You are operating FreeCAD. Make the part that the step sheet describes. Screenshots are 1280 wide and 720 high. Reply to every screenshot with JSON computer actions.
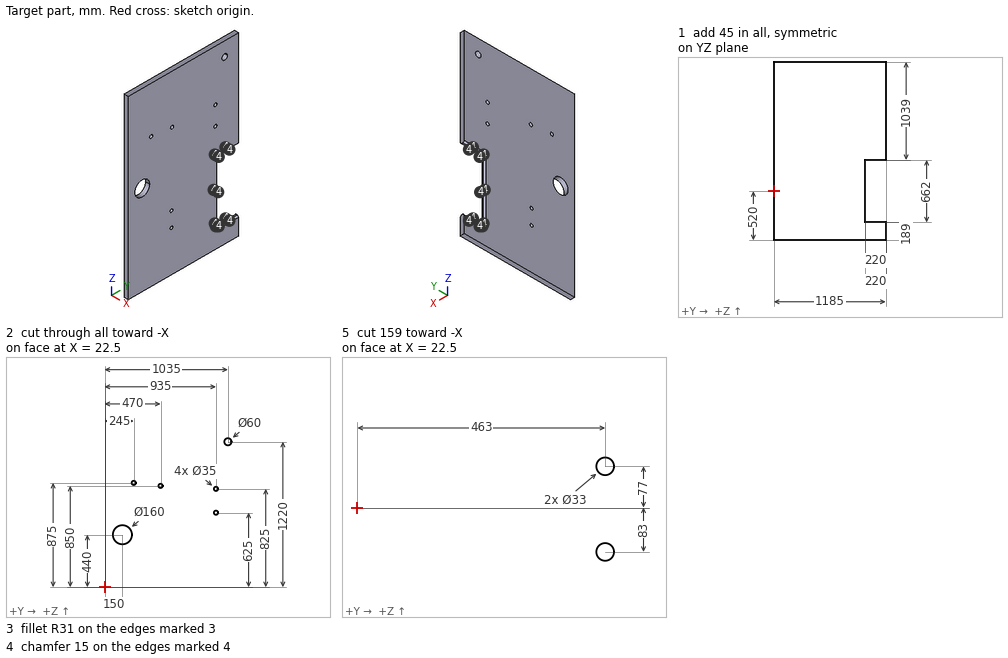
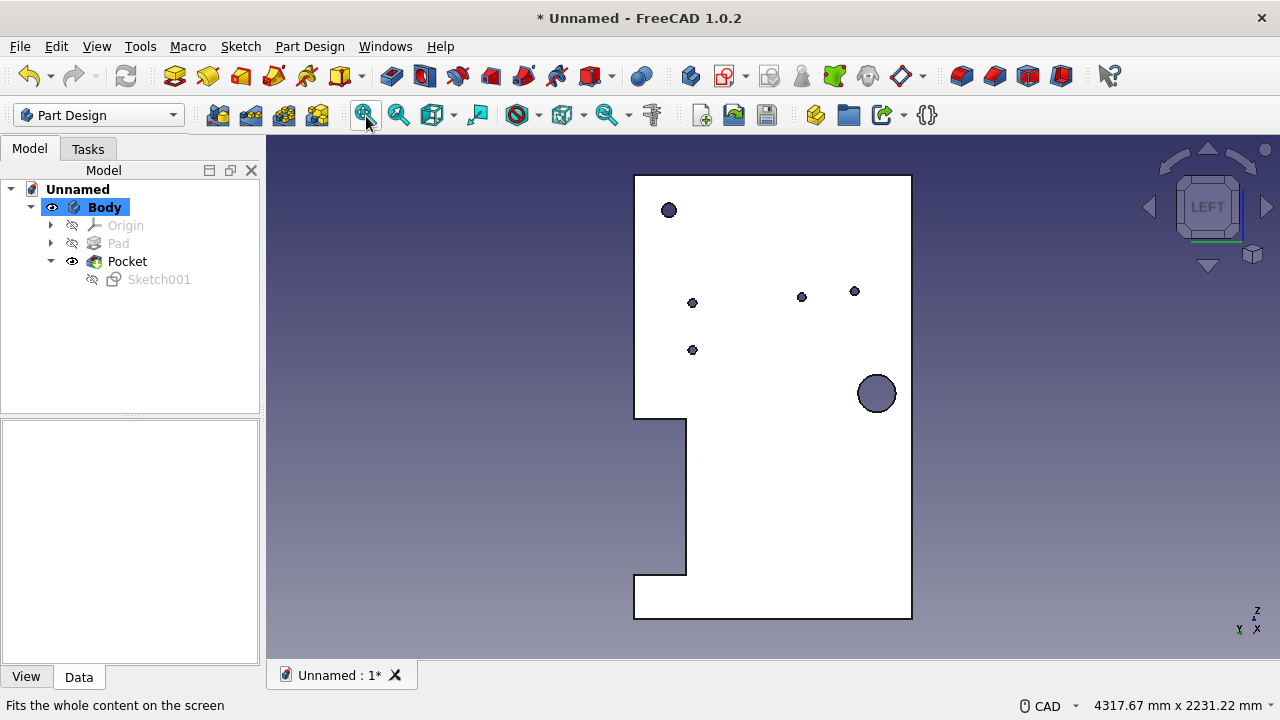
{"action": "scroll", "coordinate": [686, 418], "scroll_direction": "up", "scroll_amount": 7}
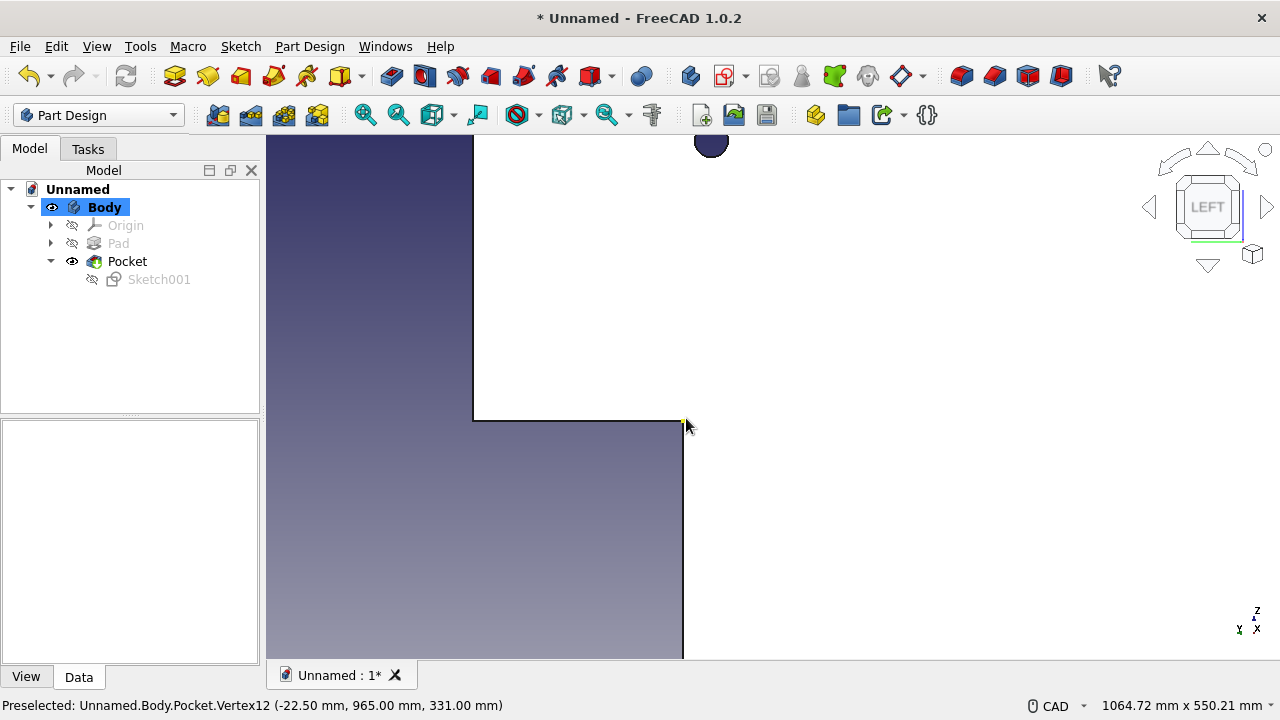
{"action": "left_click", "coordinate": [366, 116]}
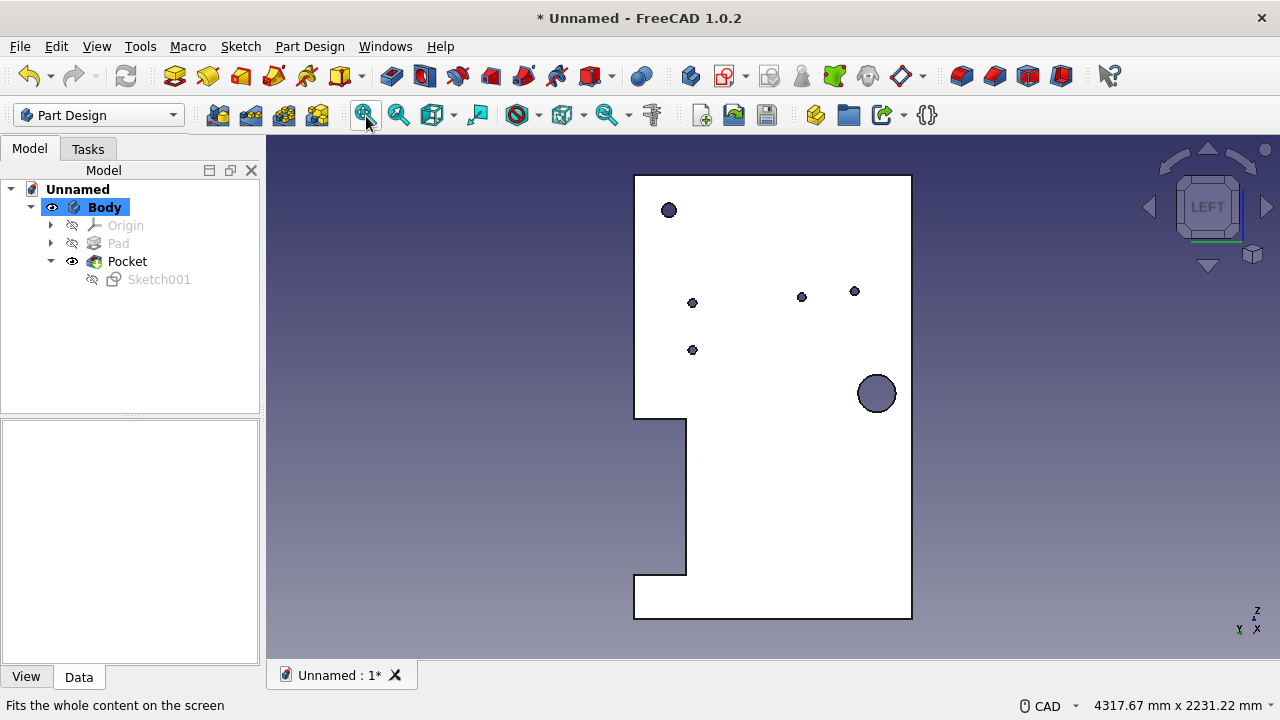
{"action": "key", "text": "v 3"}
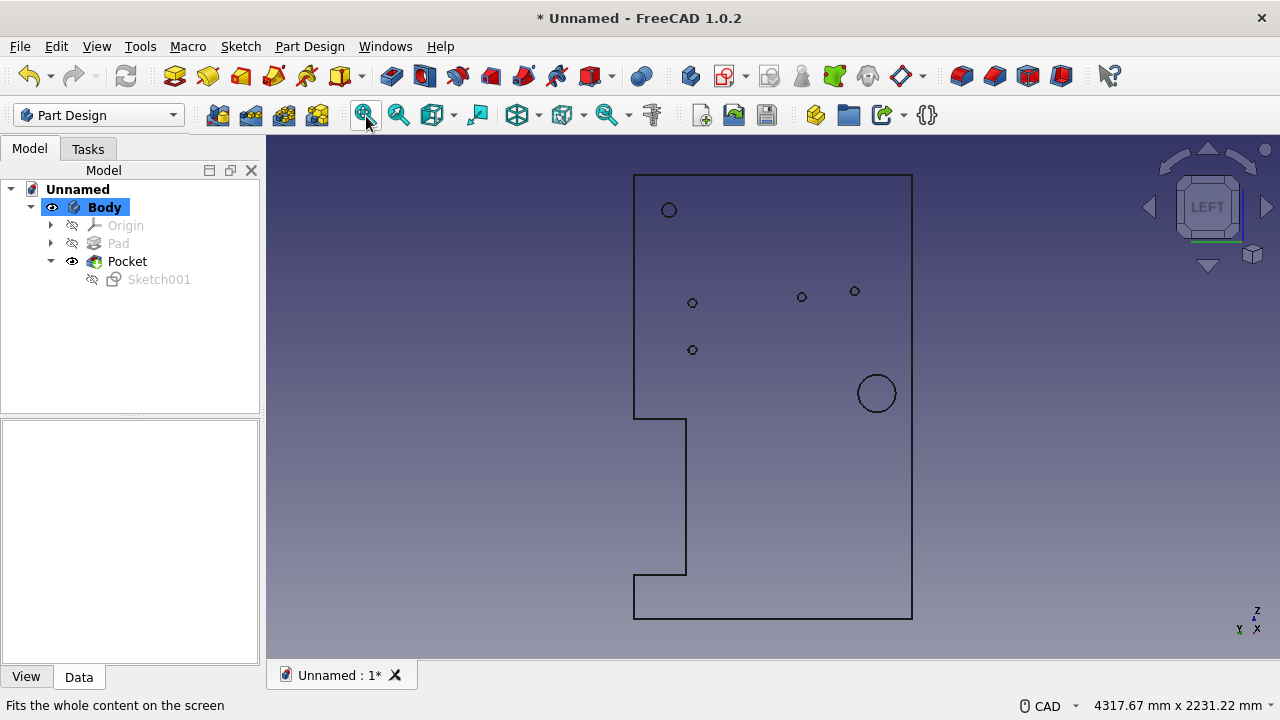
{"action": "key", "text": "0"}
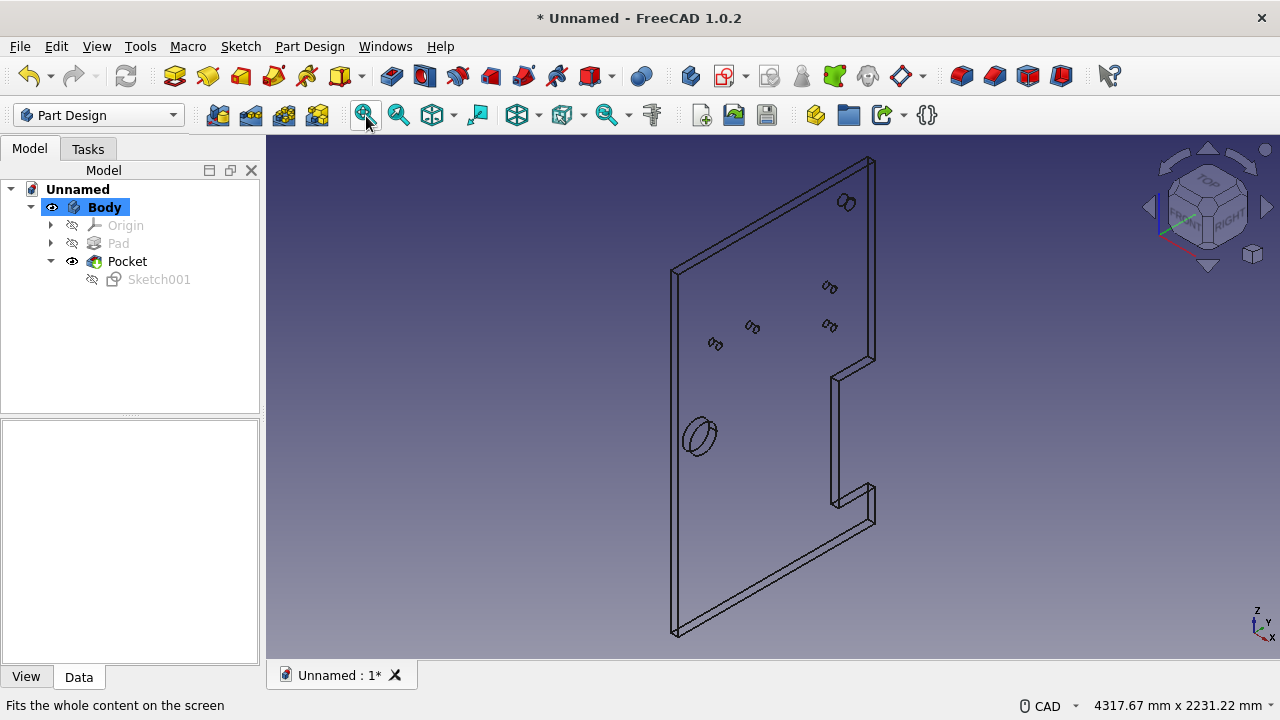
{"action": "left_click", "coordinate": [833, 377]}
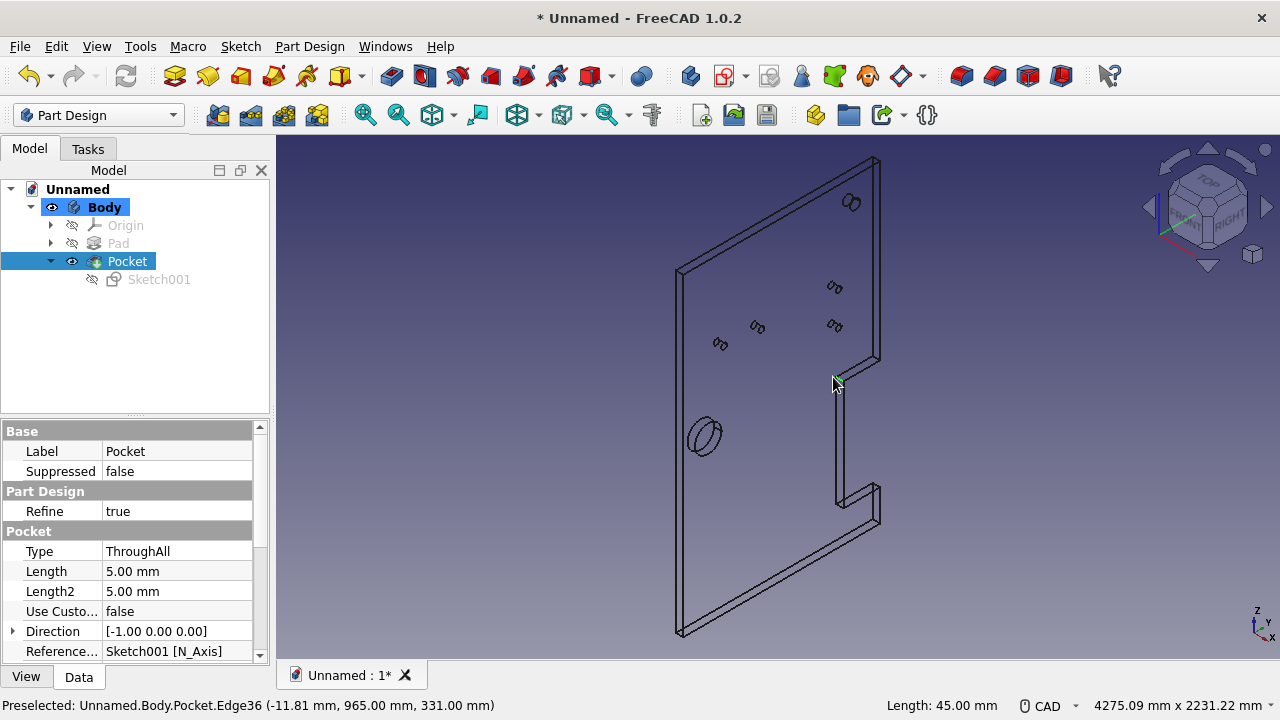
{"action": "scroll", "coordinate": [840, 505], "scroll_direction": "up", "scroll_amount": 7}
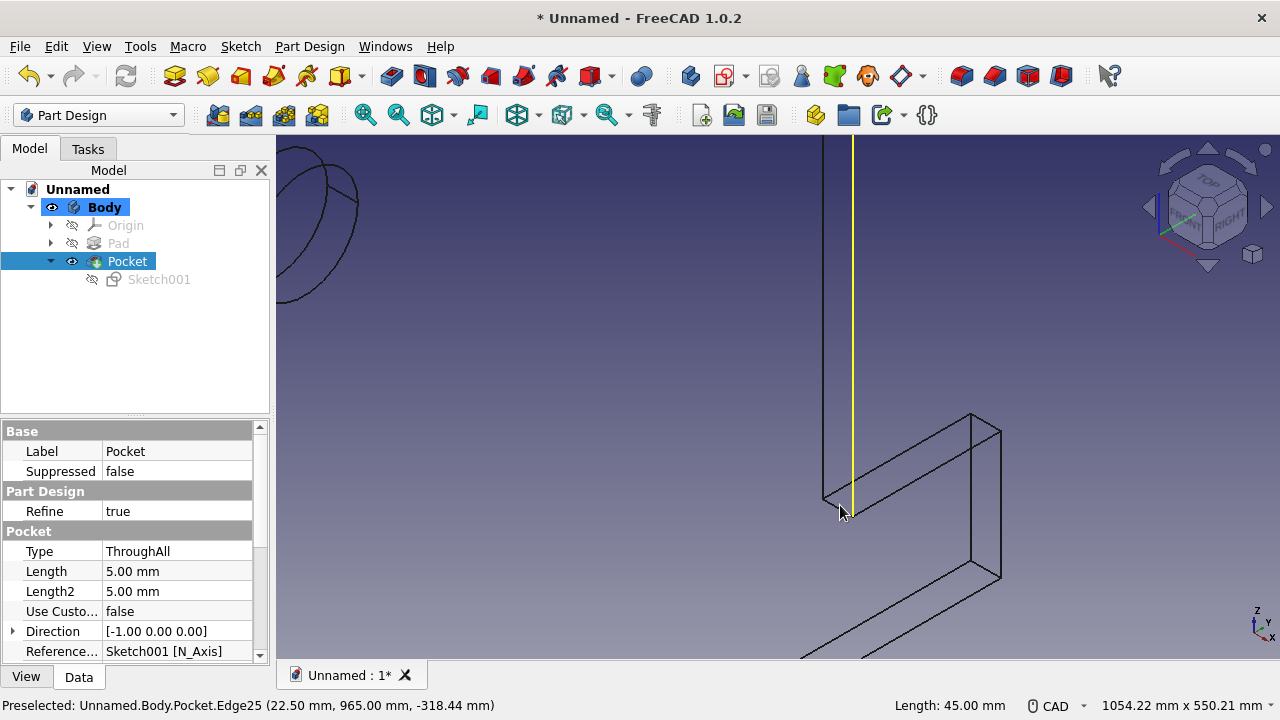
{"action": "left_click", "coordinate": [838, 507], "text": "ctrl"}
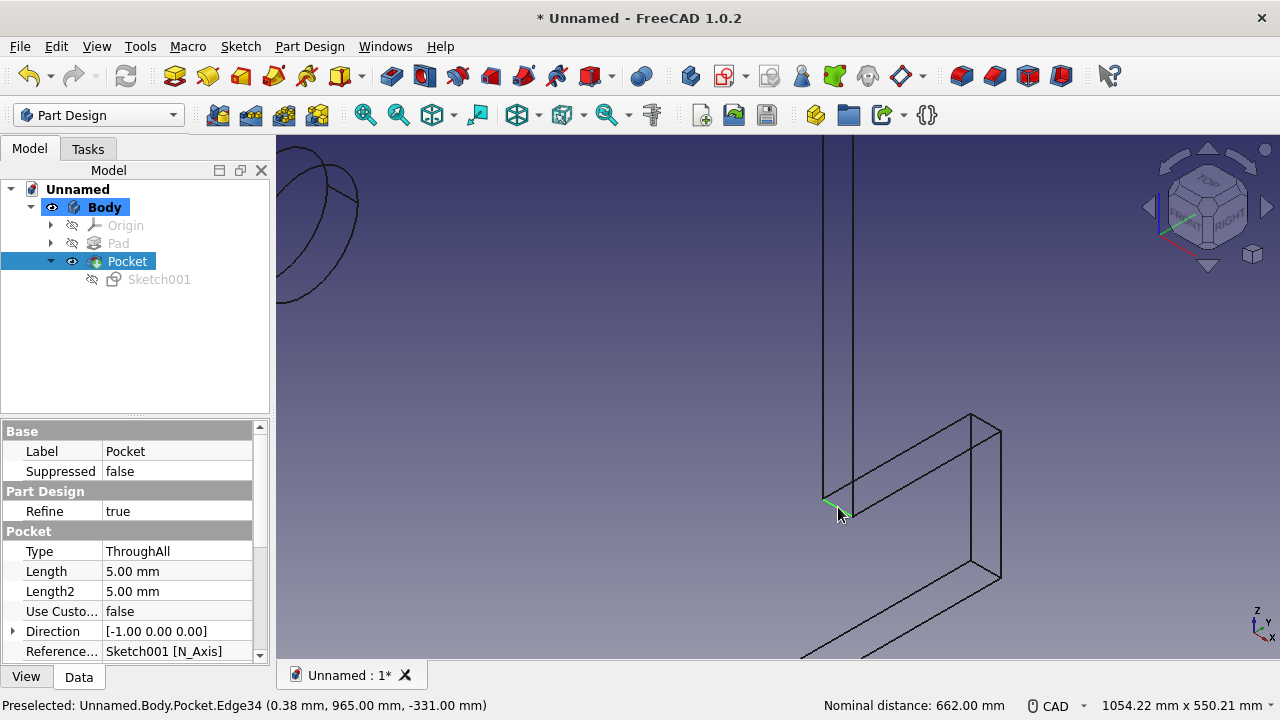
{"action": "key", "text": "v 1"}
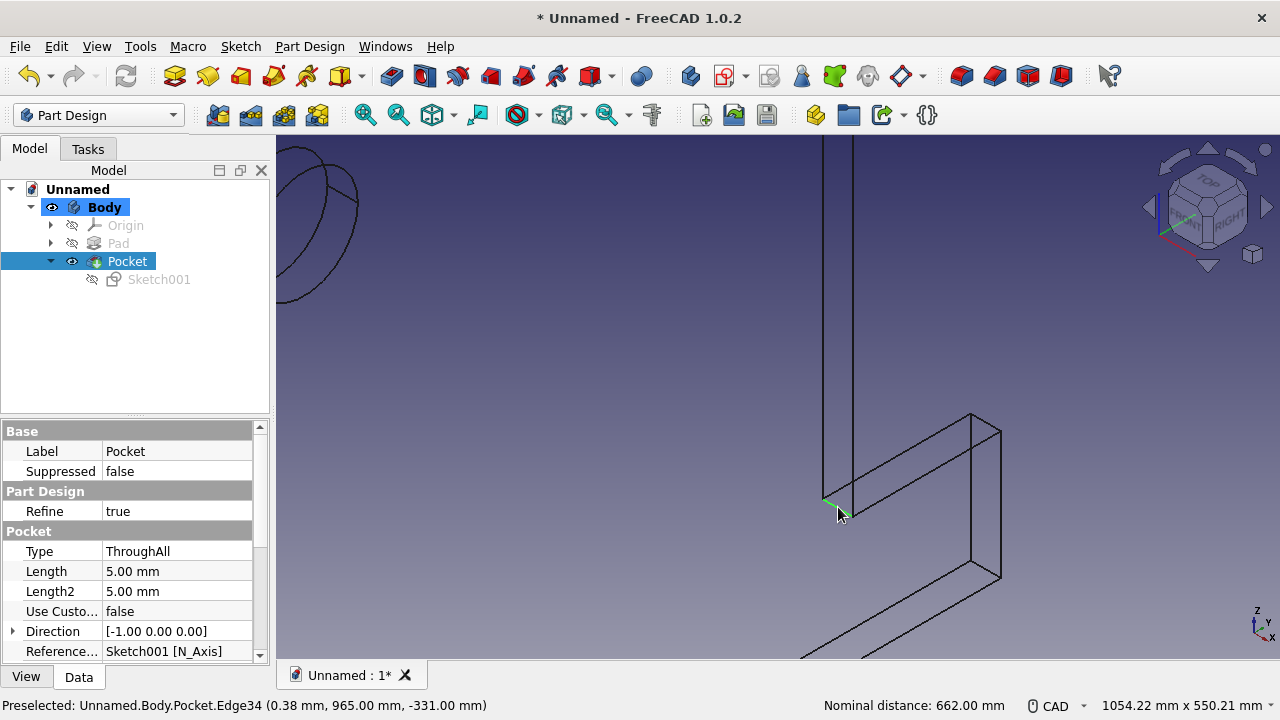
{"action": "left_click", "coordinate": [962, 76]}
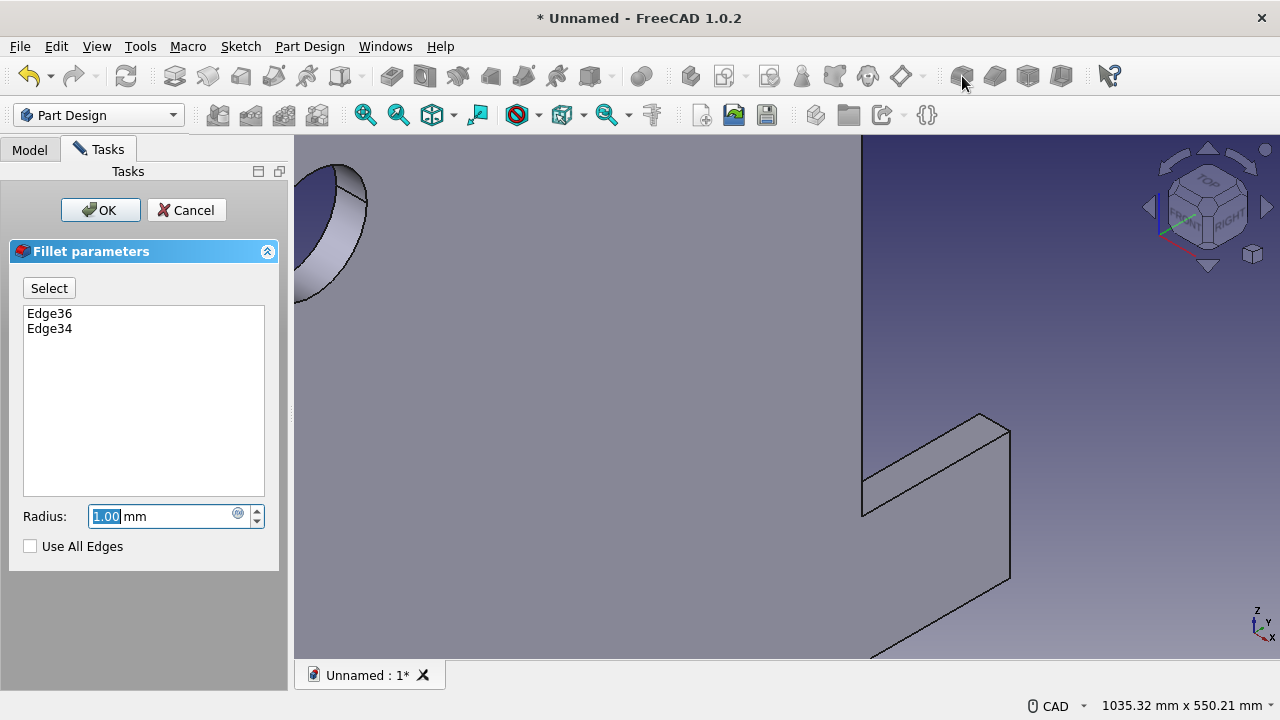
{"action": "type", "text": "31"}
{"action": "key", "text": "Tab"}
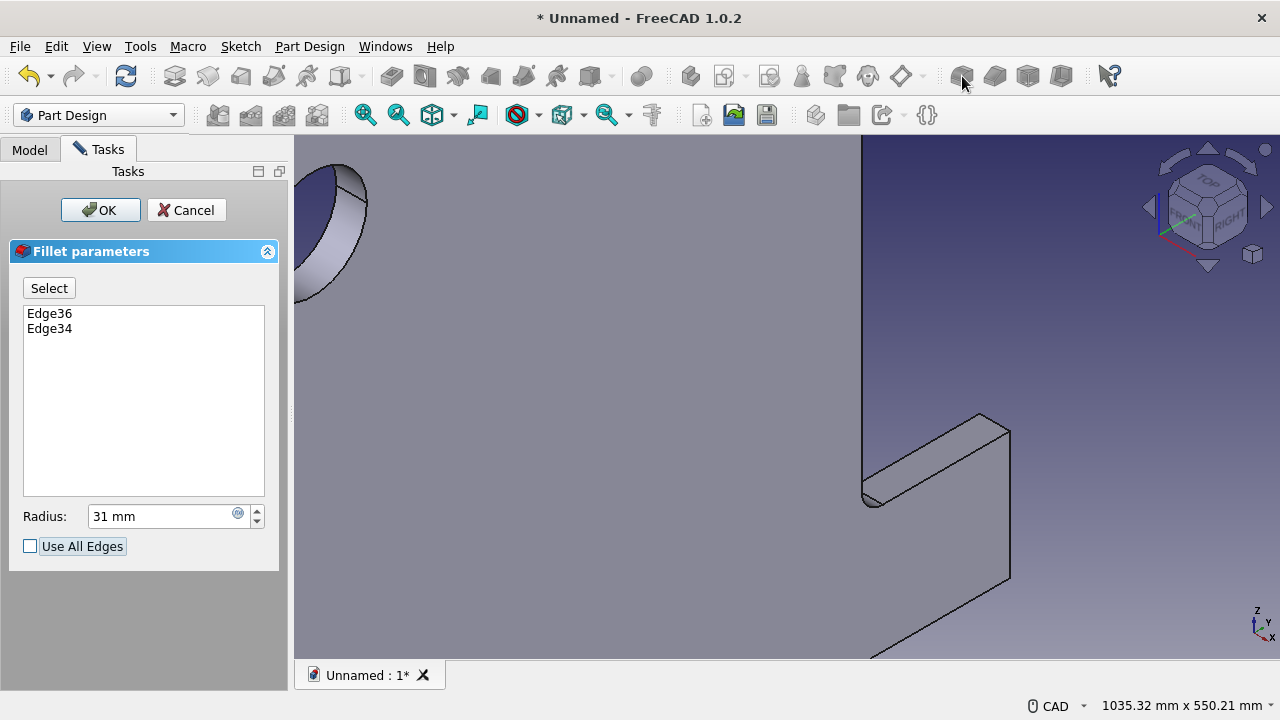
{"action": "left_click", "coordinate": [101, 210]}